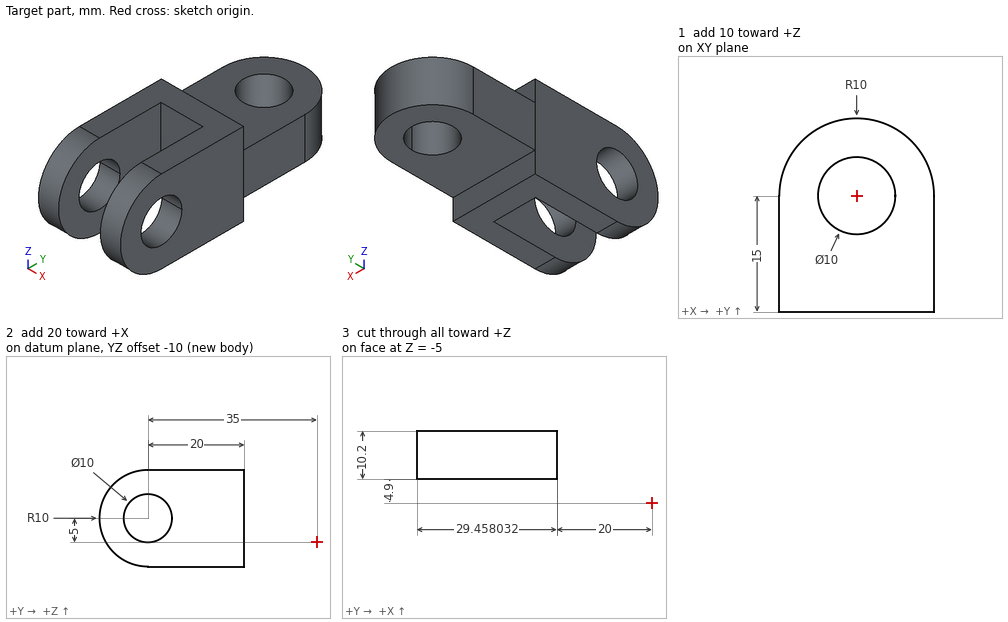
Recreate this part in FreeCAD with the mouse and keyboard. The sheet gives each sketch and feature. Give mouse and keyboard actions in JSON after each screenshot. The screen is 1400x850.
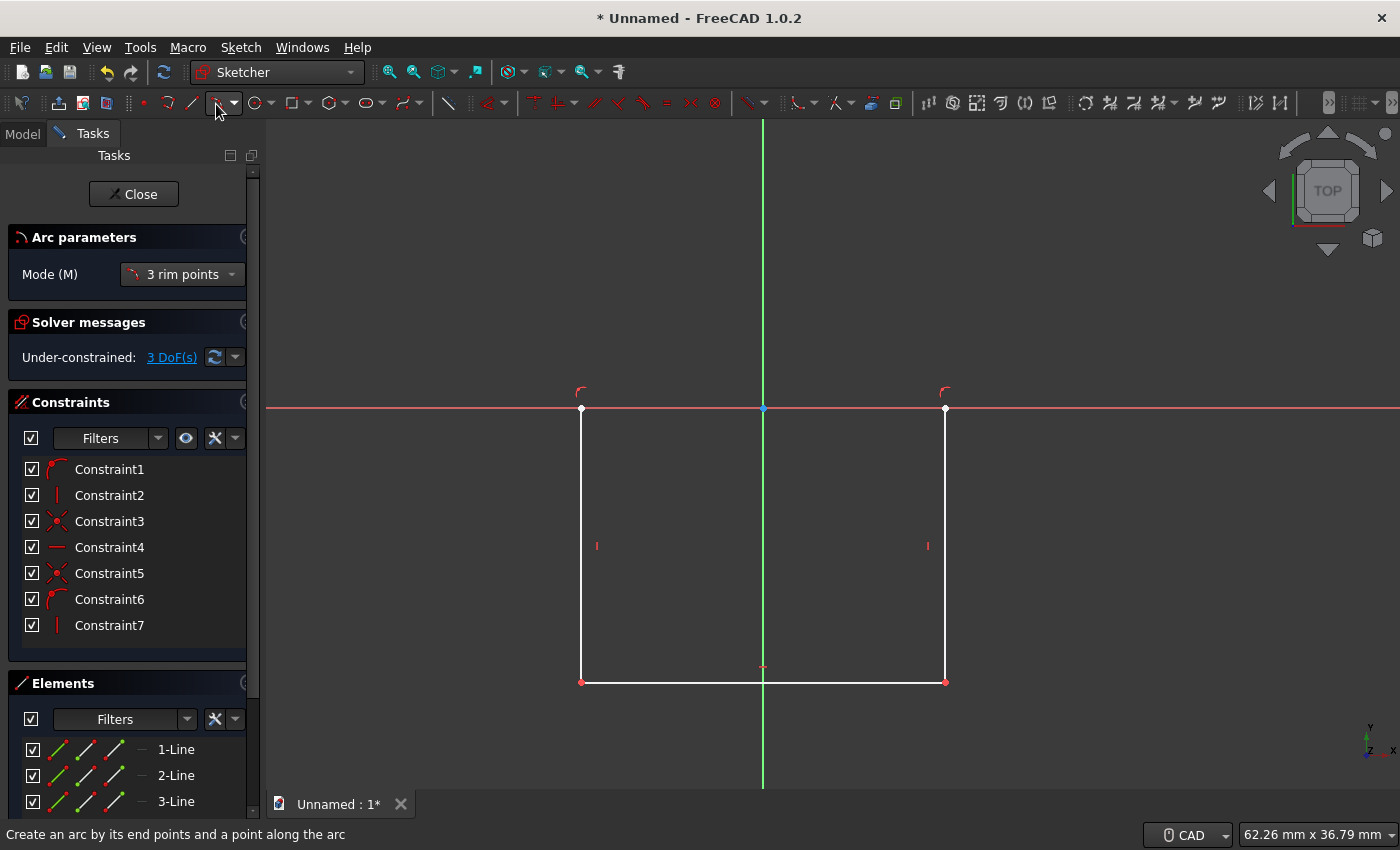
{"action": "left_click", "coordinate": [945, 408]}
{"action": "left_click", "coordinate": [581, 408]}
{"action": "left_click", "coordinate": [820, 235]}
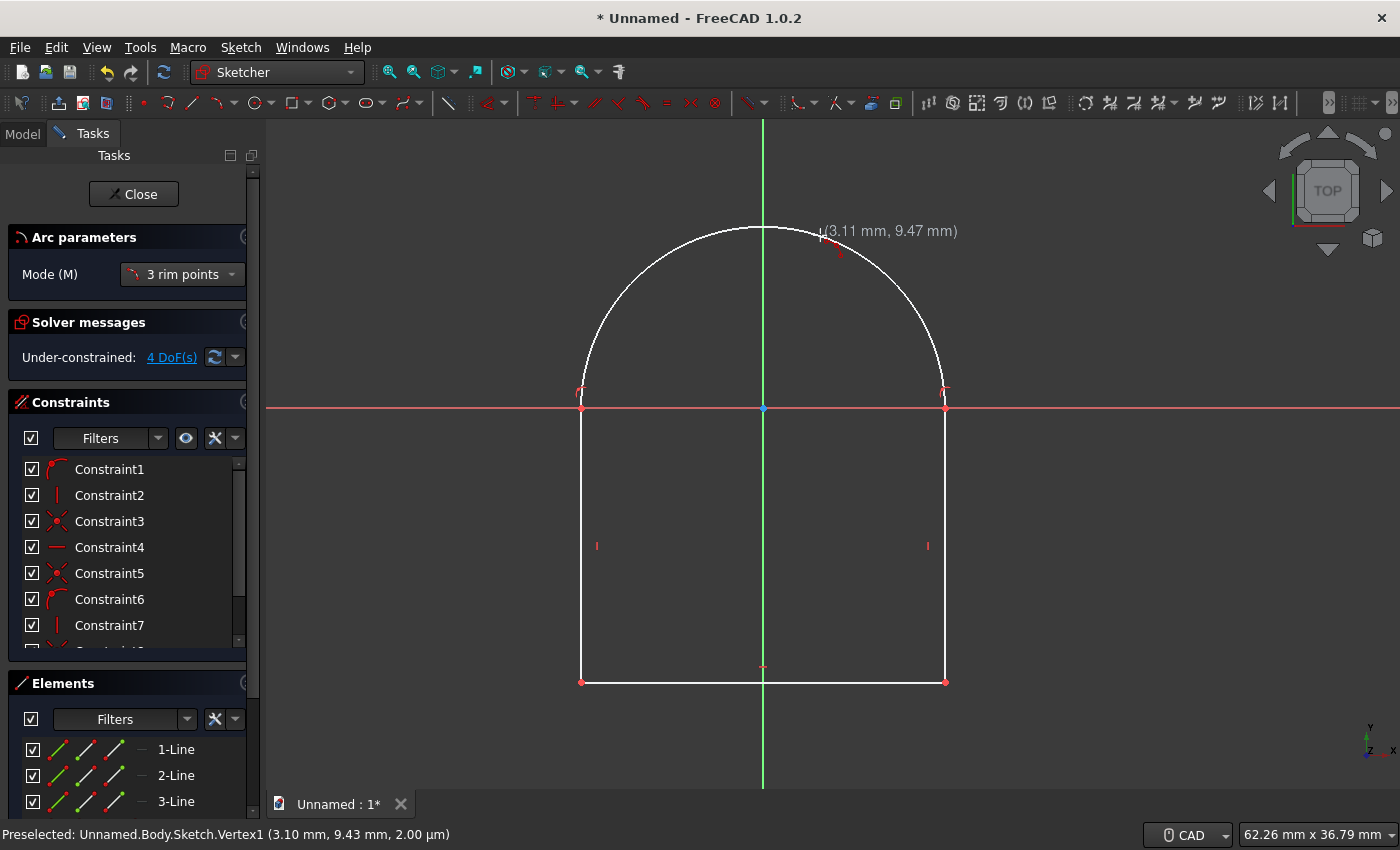
{"action": "left_click", "coordinate": [256, 104]}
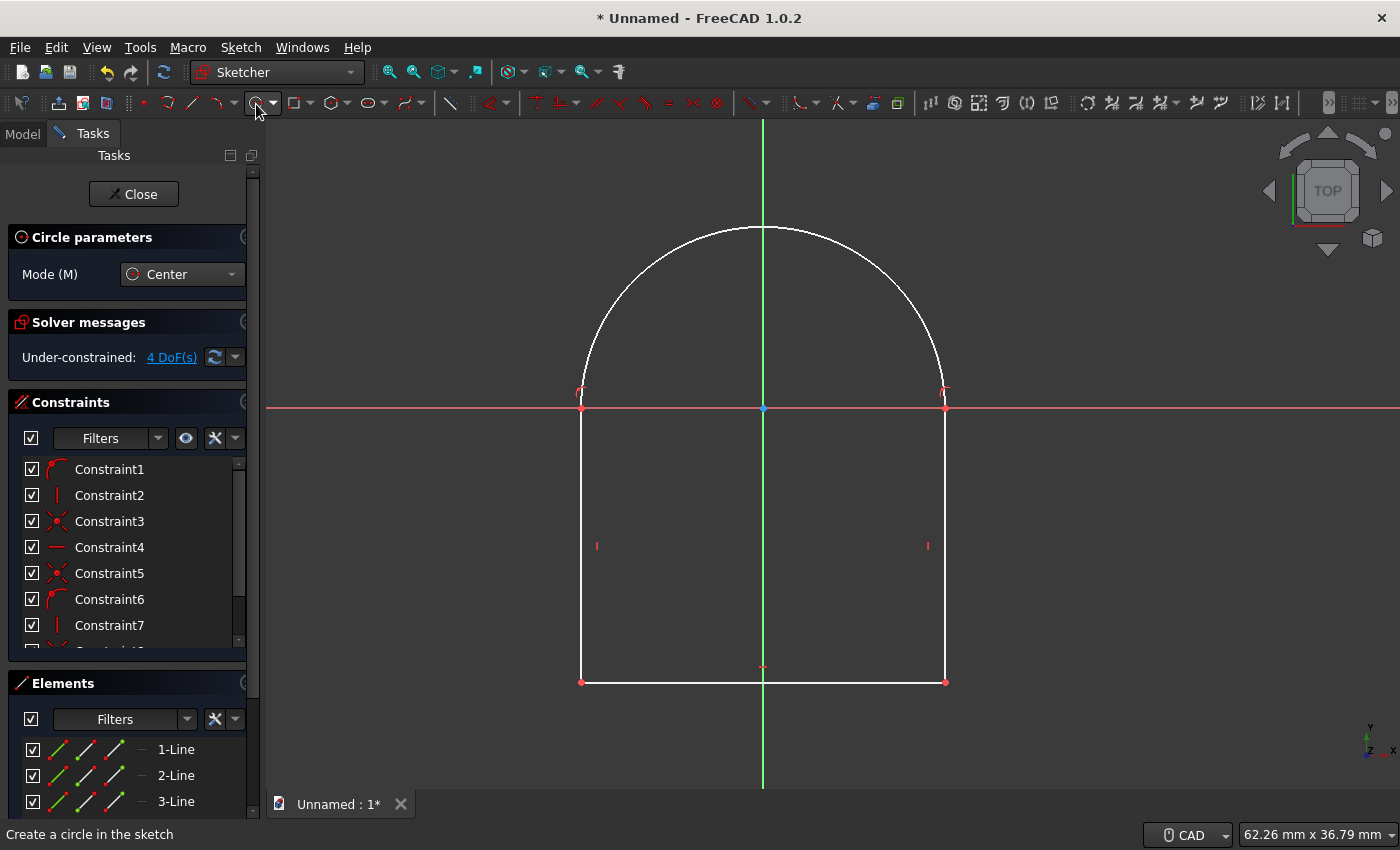
{"action": "left_click", "coordinate": [763, 408]}
{"action": "left_click", "coordinate": [828, 344]}
{"action": "key", "text": "Escape"}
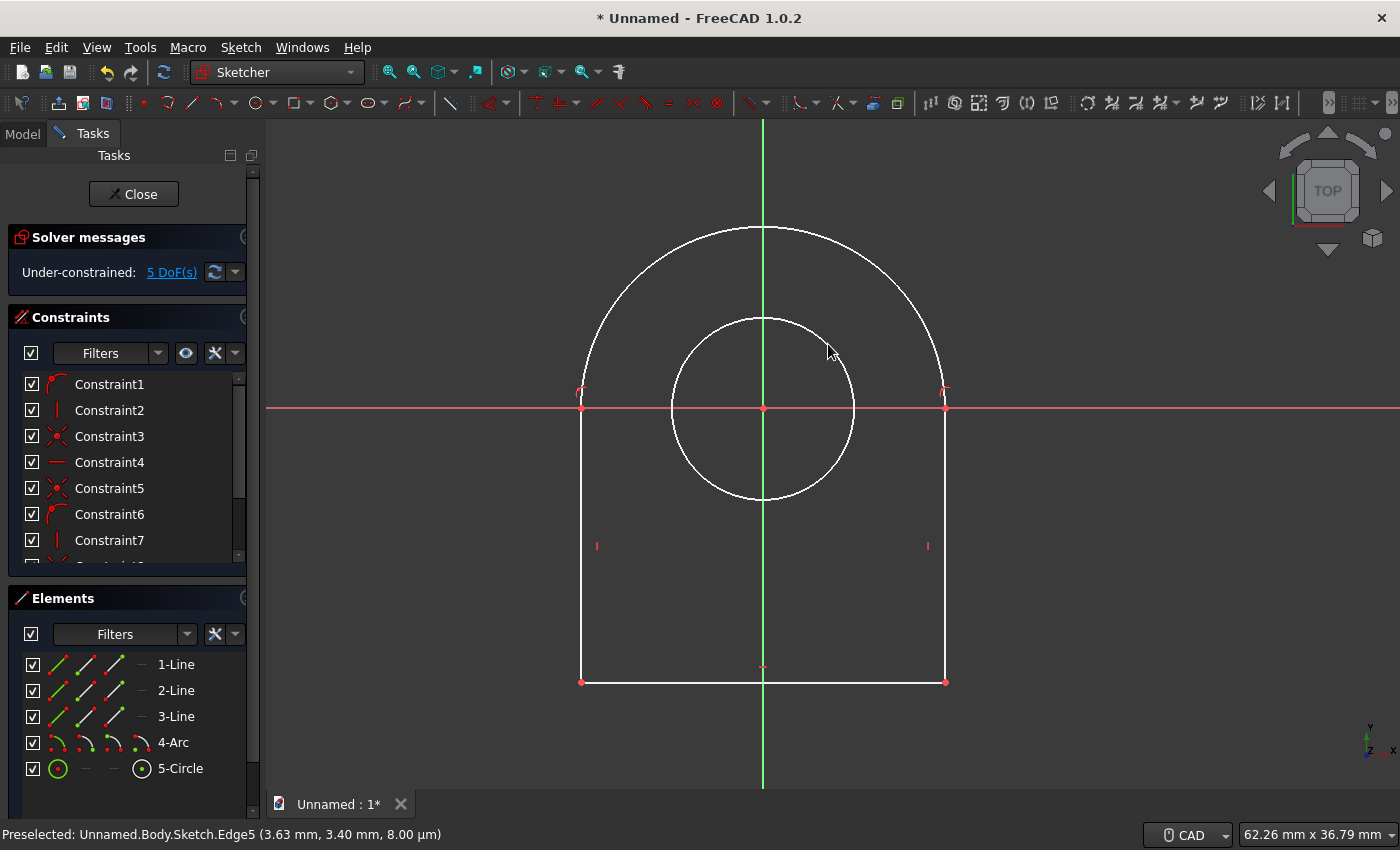
{"action": "left_click", "coordinate": [581, 491]}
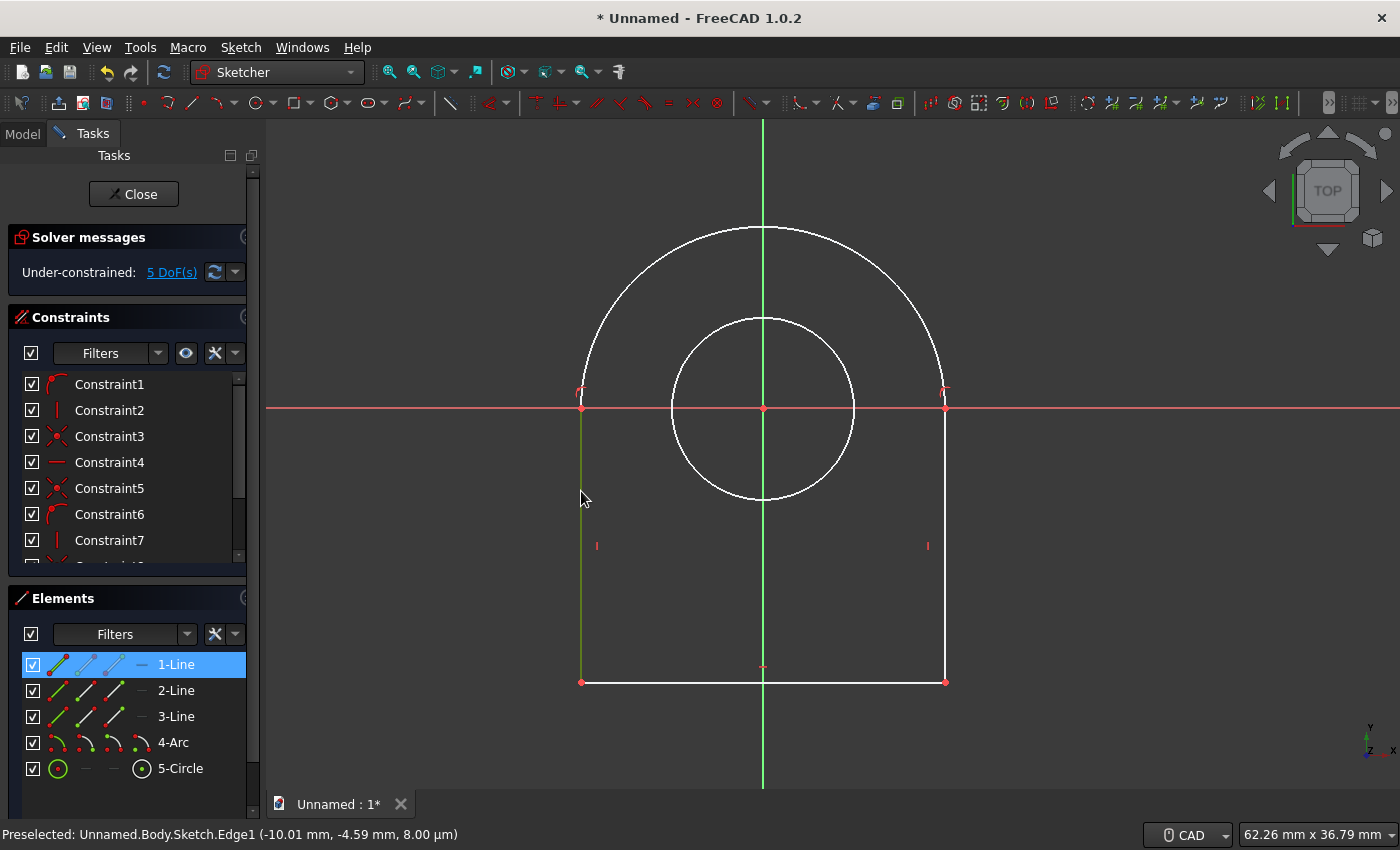
{"action": "left_click", "coordinate": [870, 261]}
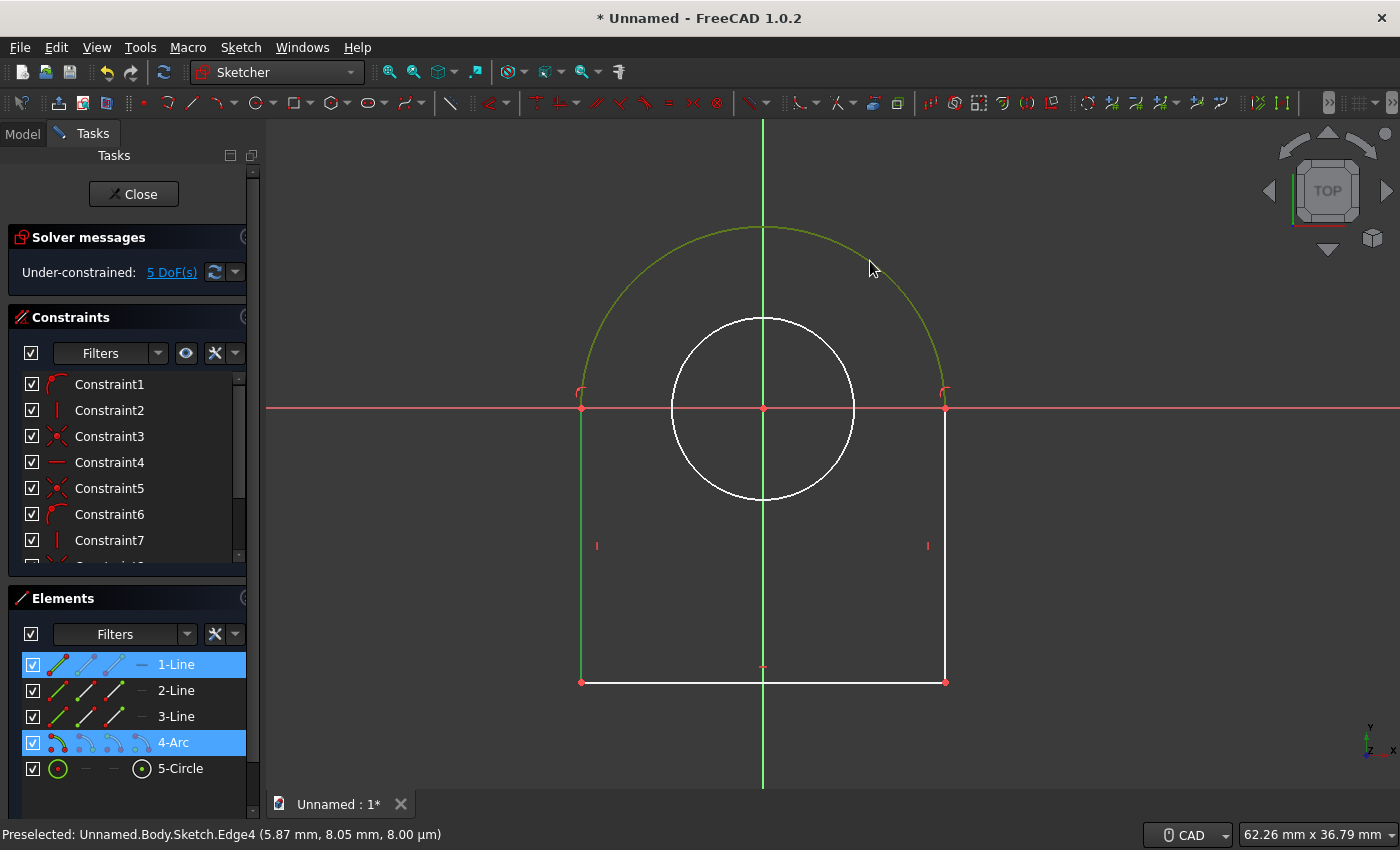
{"action": "left_click", "coordinate": [646, 104]}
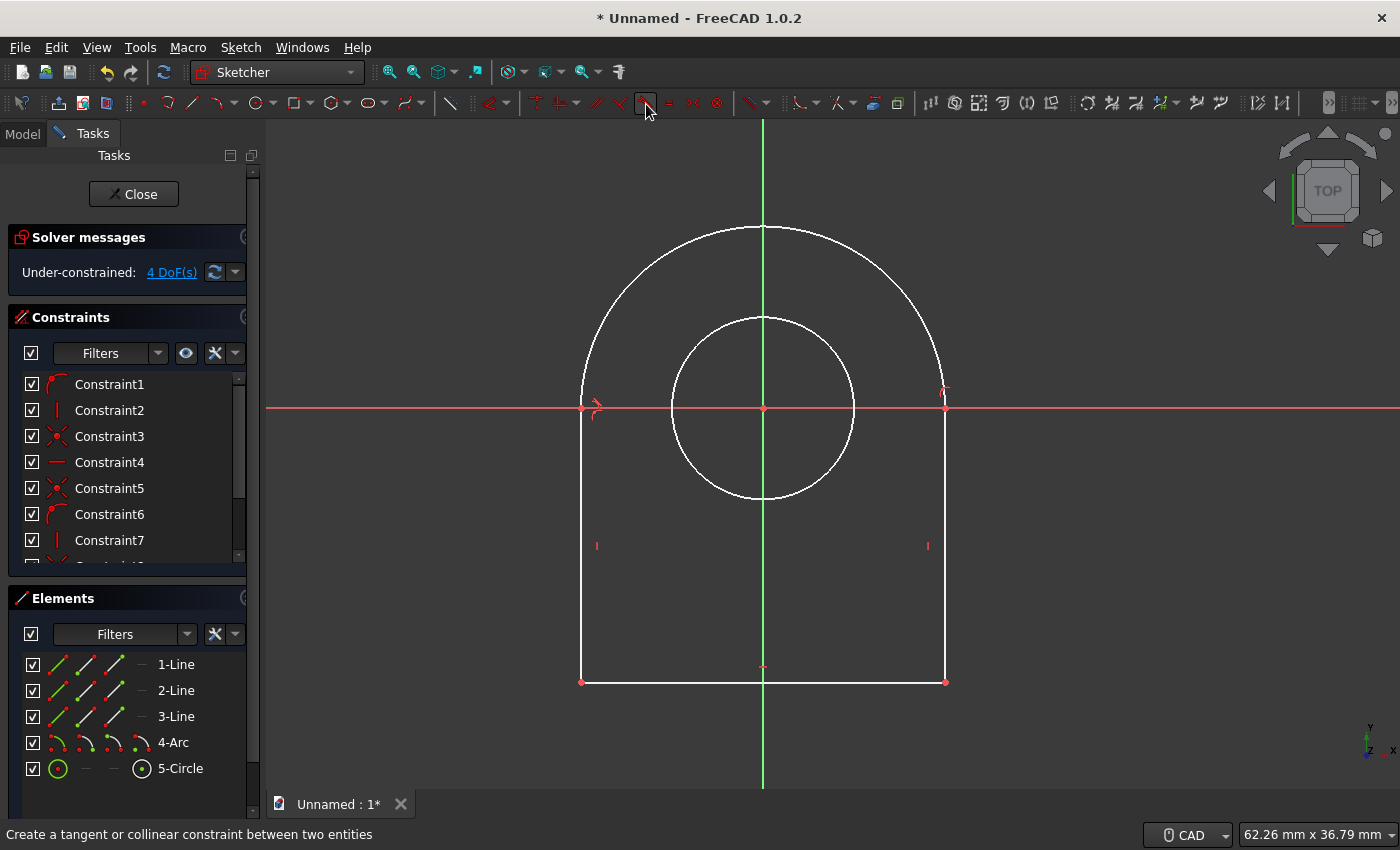
{"action": "left_click", "coordinate": [763, 408]}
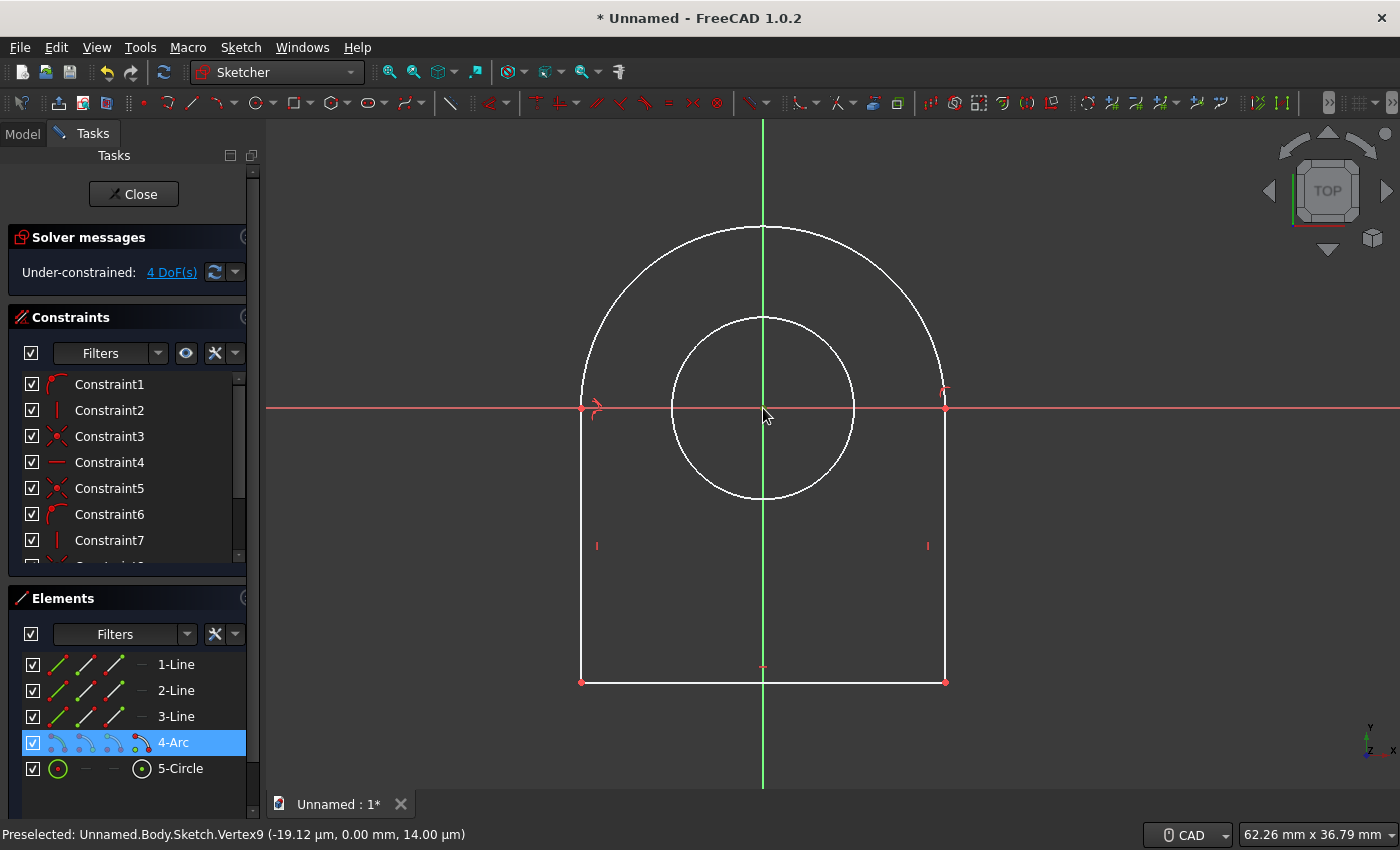
{"action": "left_click", "coordinate": [763, 717]}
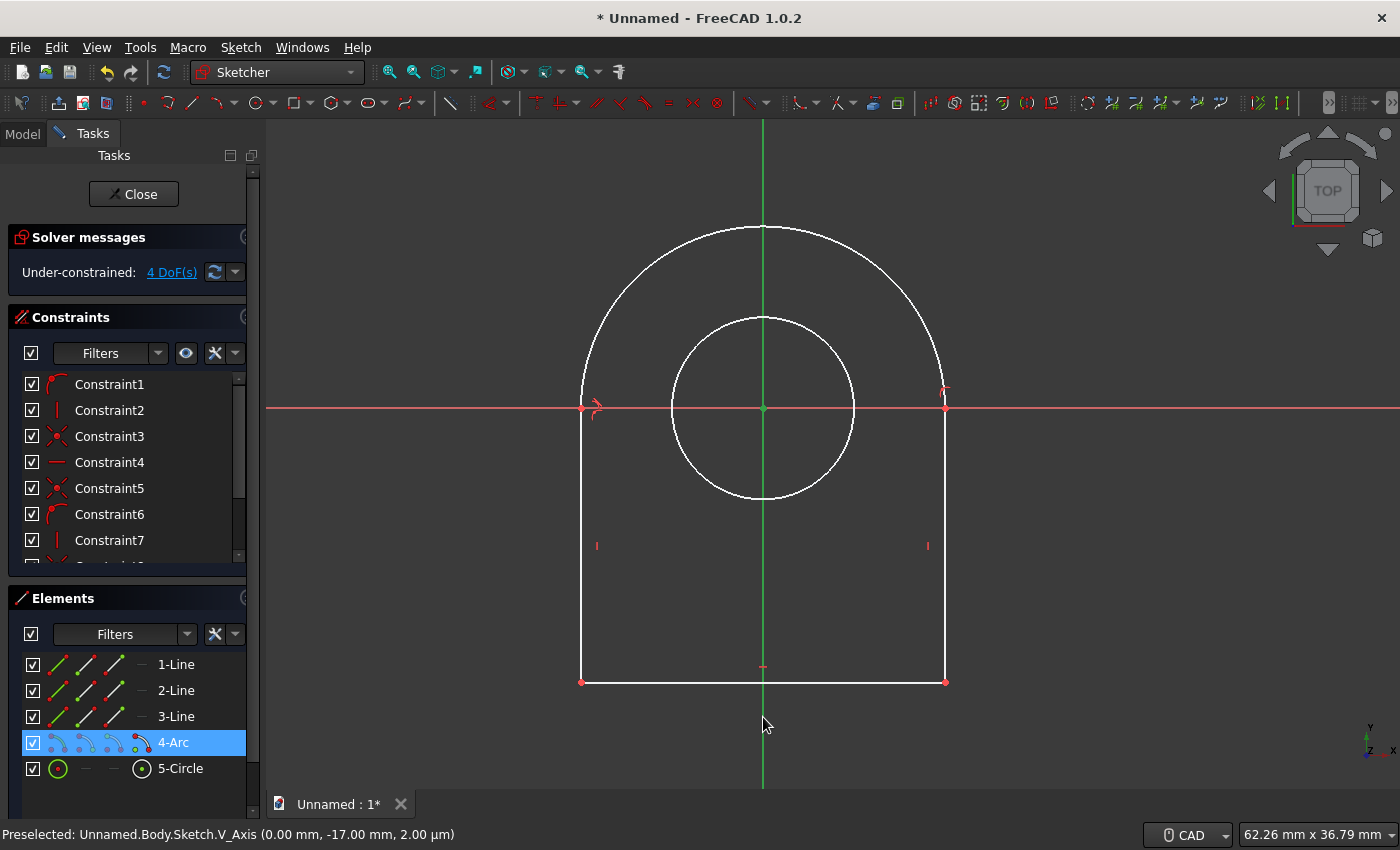
{"action": "left_click", "coordinate": [536, 104]}